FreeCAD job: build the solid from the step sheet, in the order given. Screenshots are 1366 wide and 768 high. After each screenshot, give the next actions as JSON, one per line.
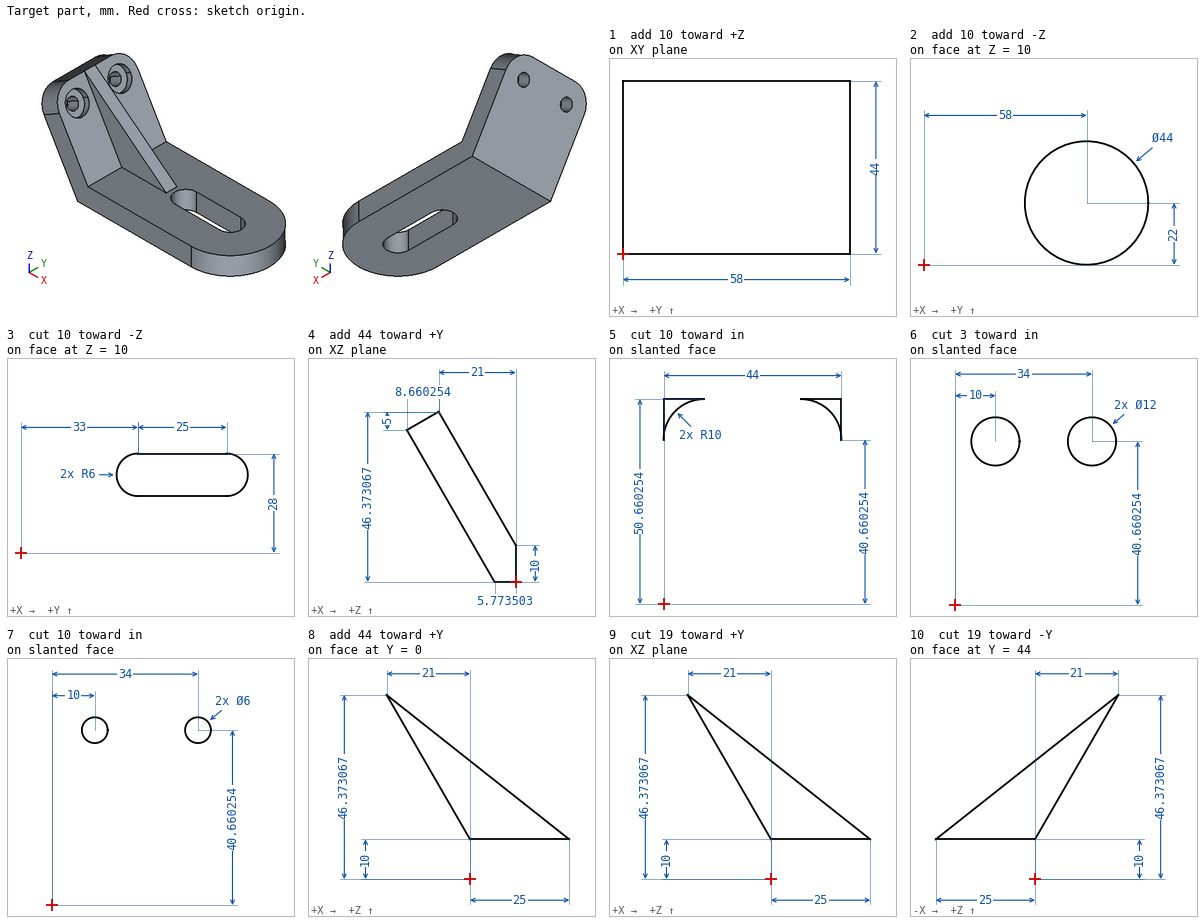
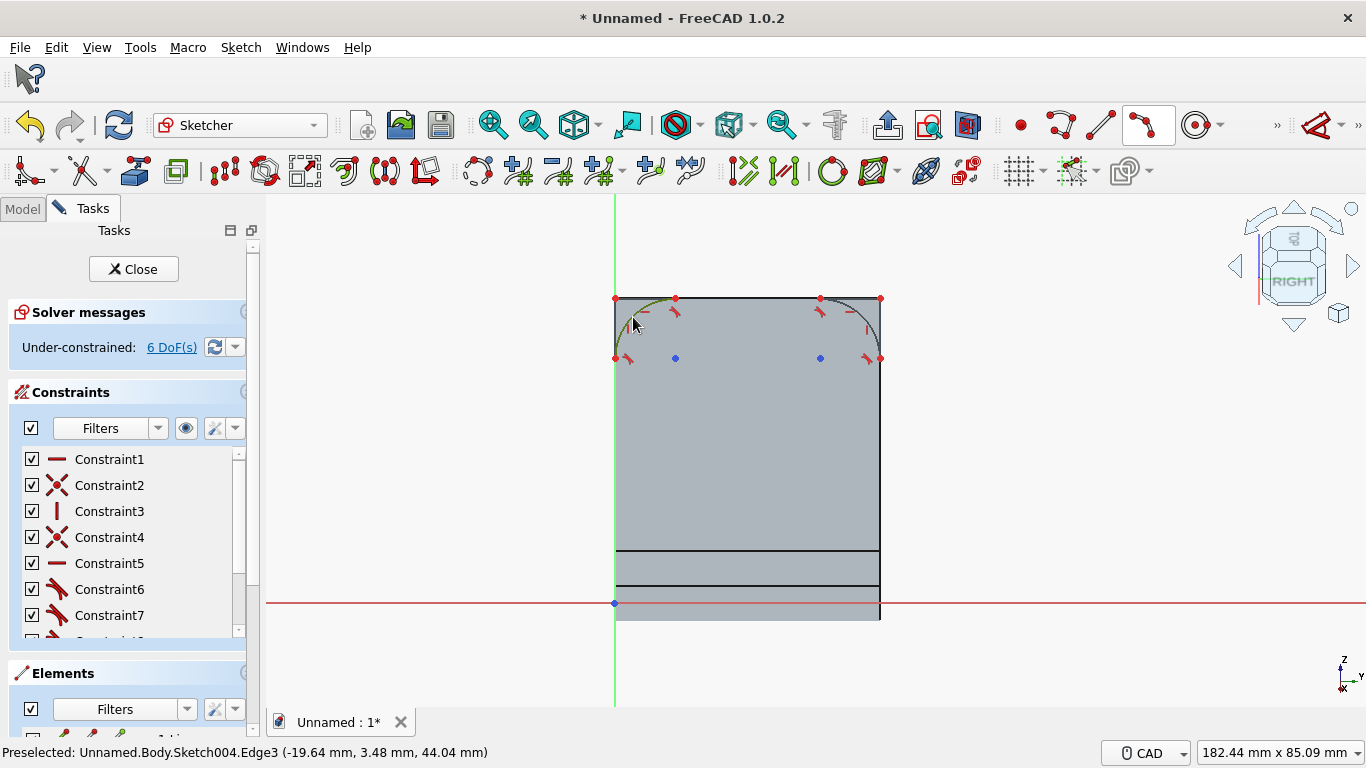
{"action": "left_click", "coordinate": [862, 317]}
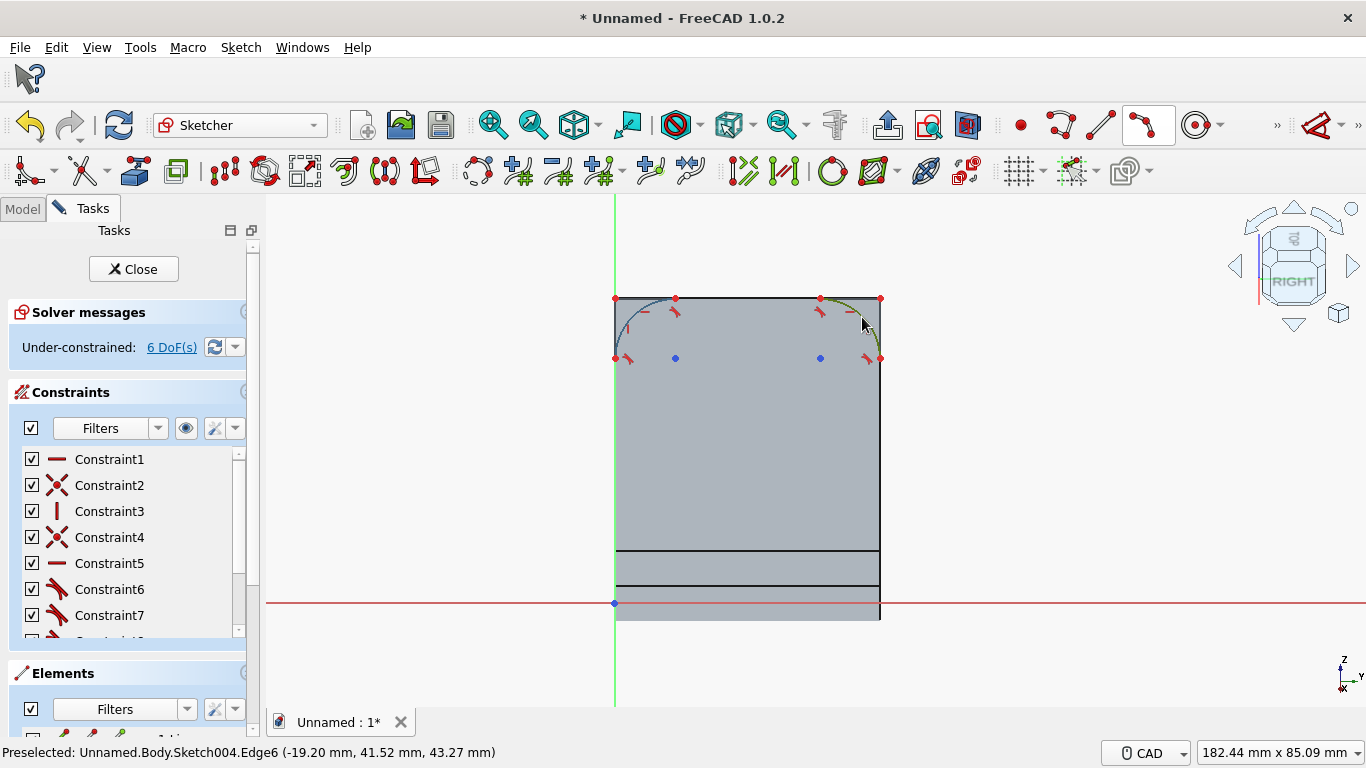
{"action": "key", "text": "e"}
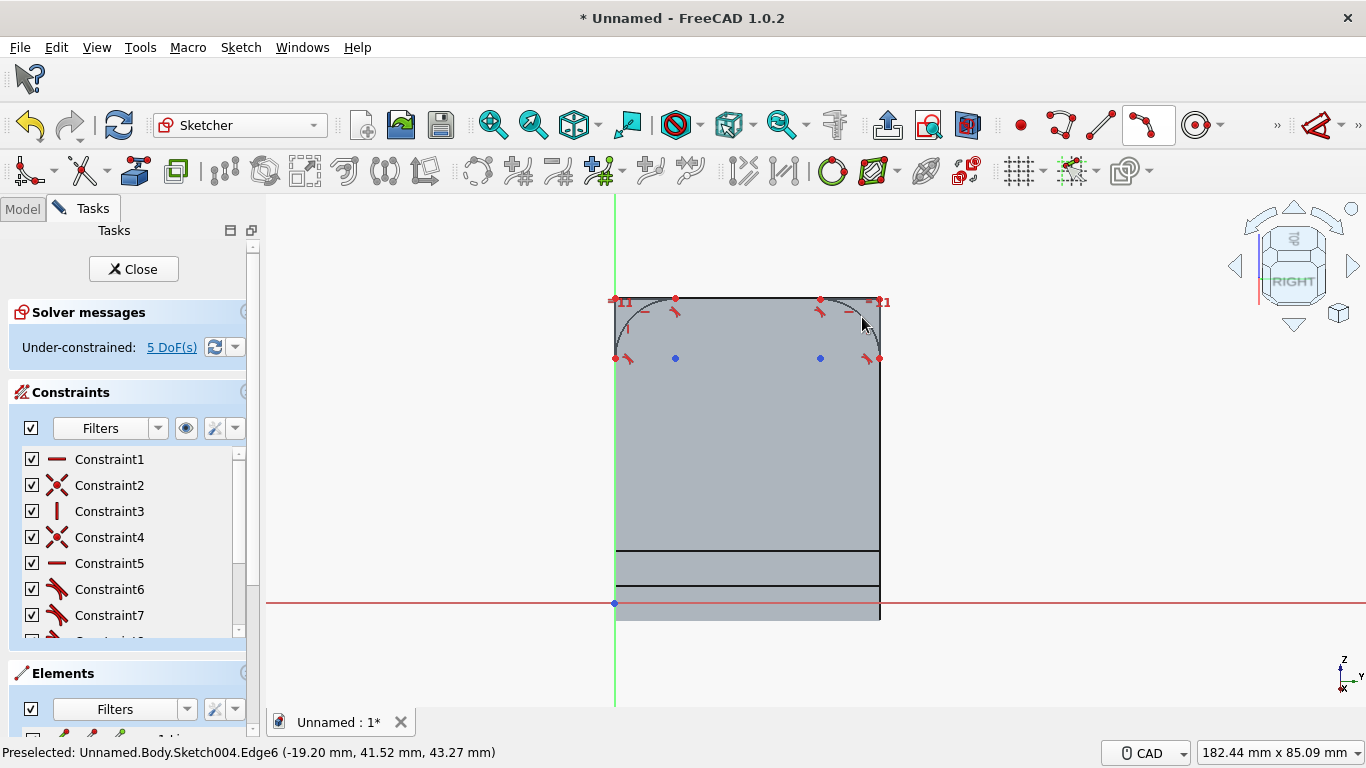
{"action": "left_click", "coordinate": [1316, 126]}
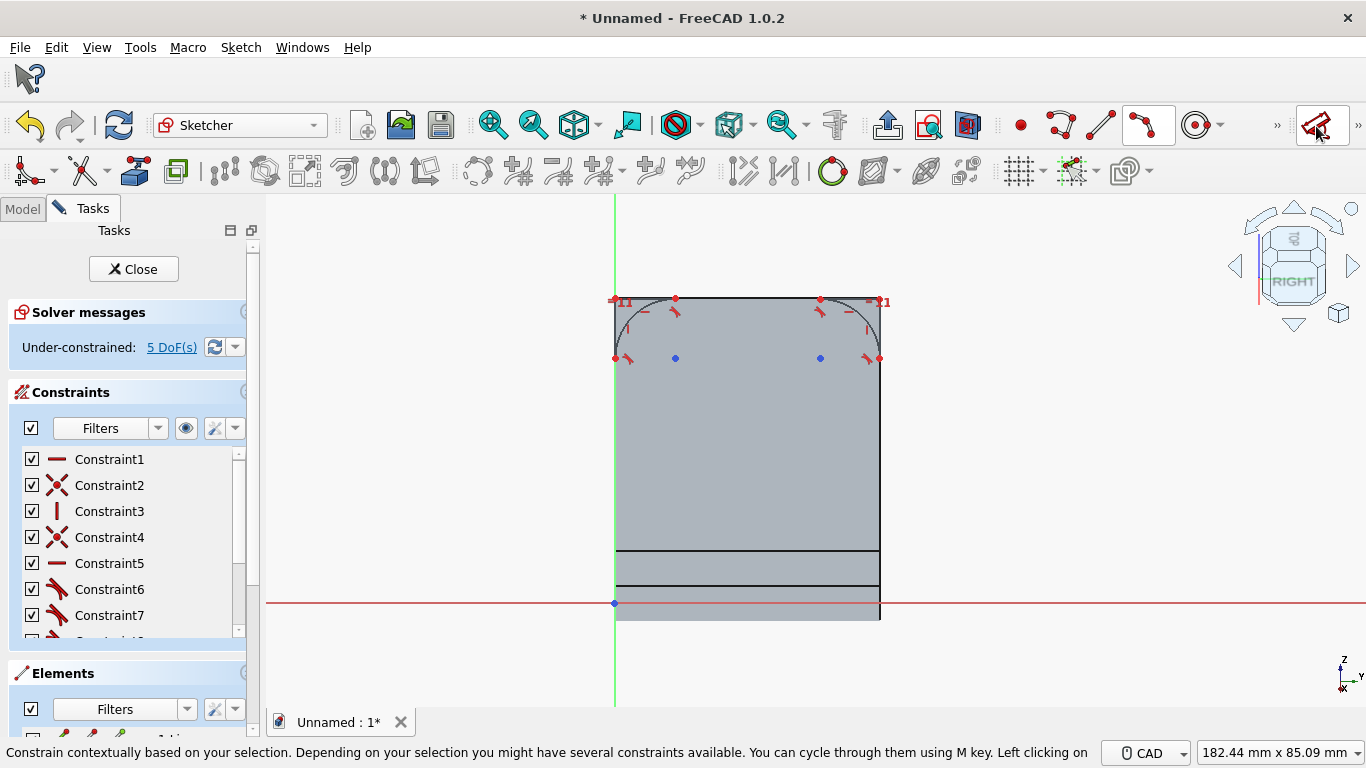
{"action": "left_click", "coordinate": [633, 317]}
{"action": "left_click", "coordinate": [649, 271]}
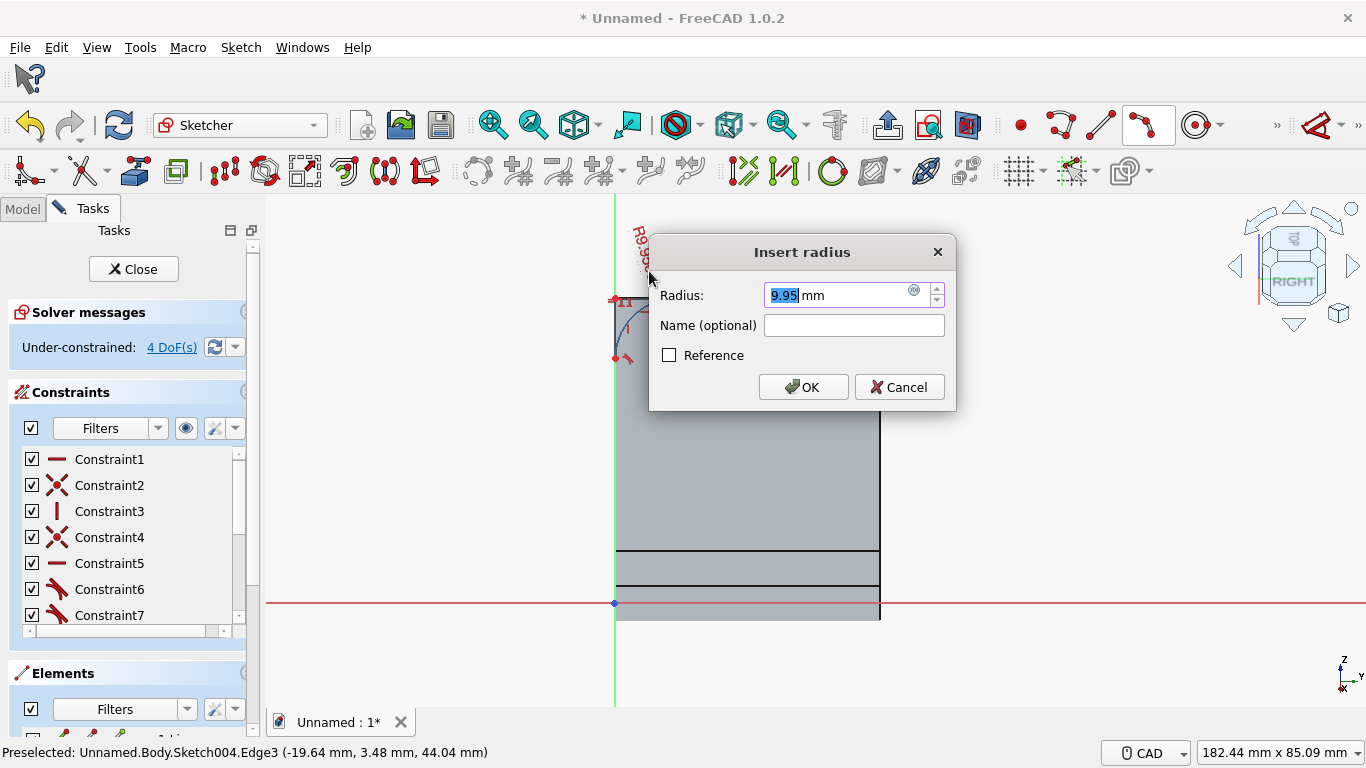
{"action": "type", "text": "10"}
{"action": "key", "text": "Return"}
{"action": "key", "text": "Escape"}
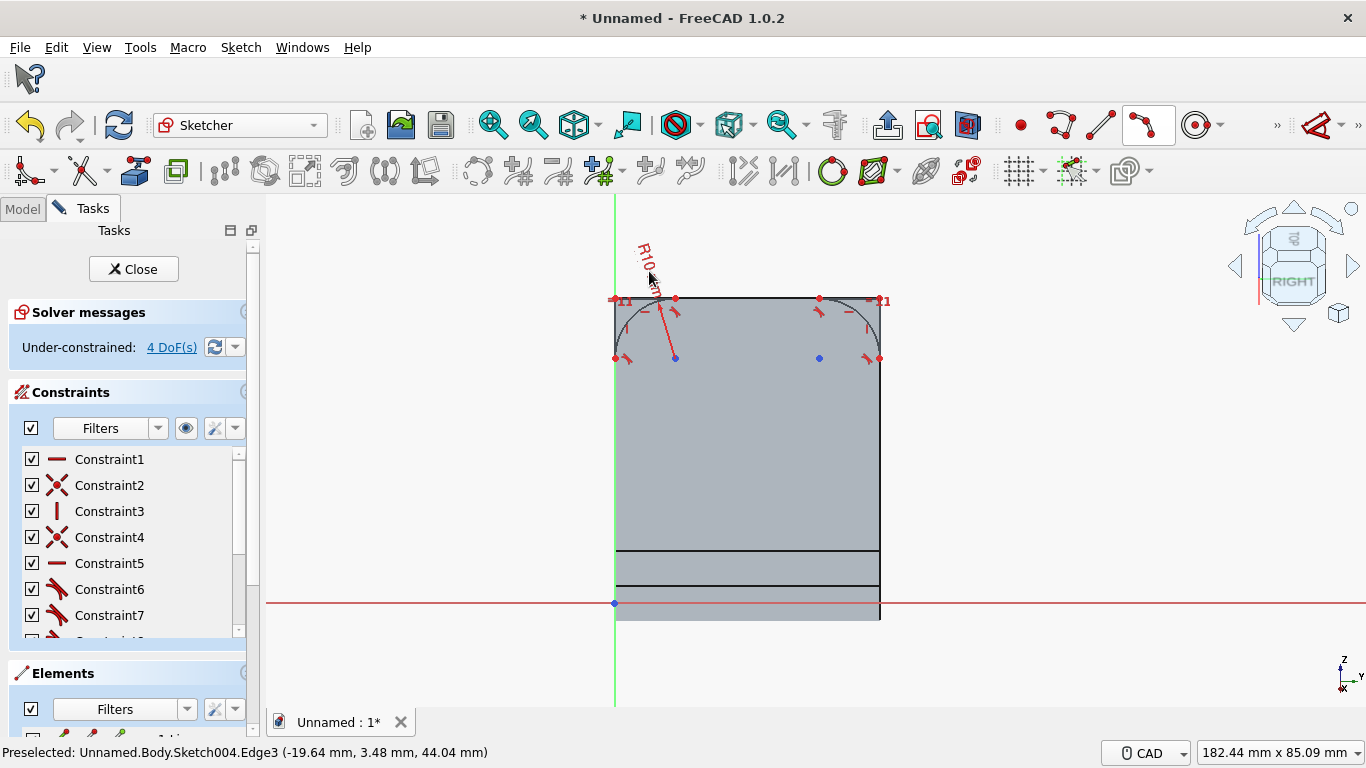
{"action": "left_click", "coordinate": [615, 299]}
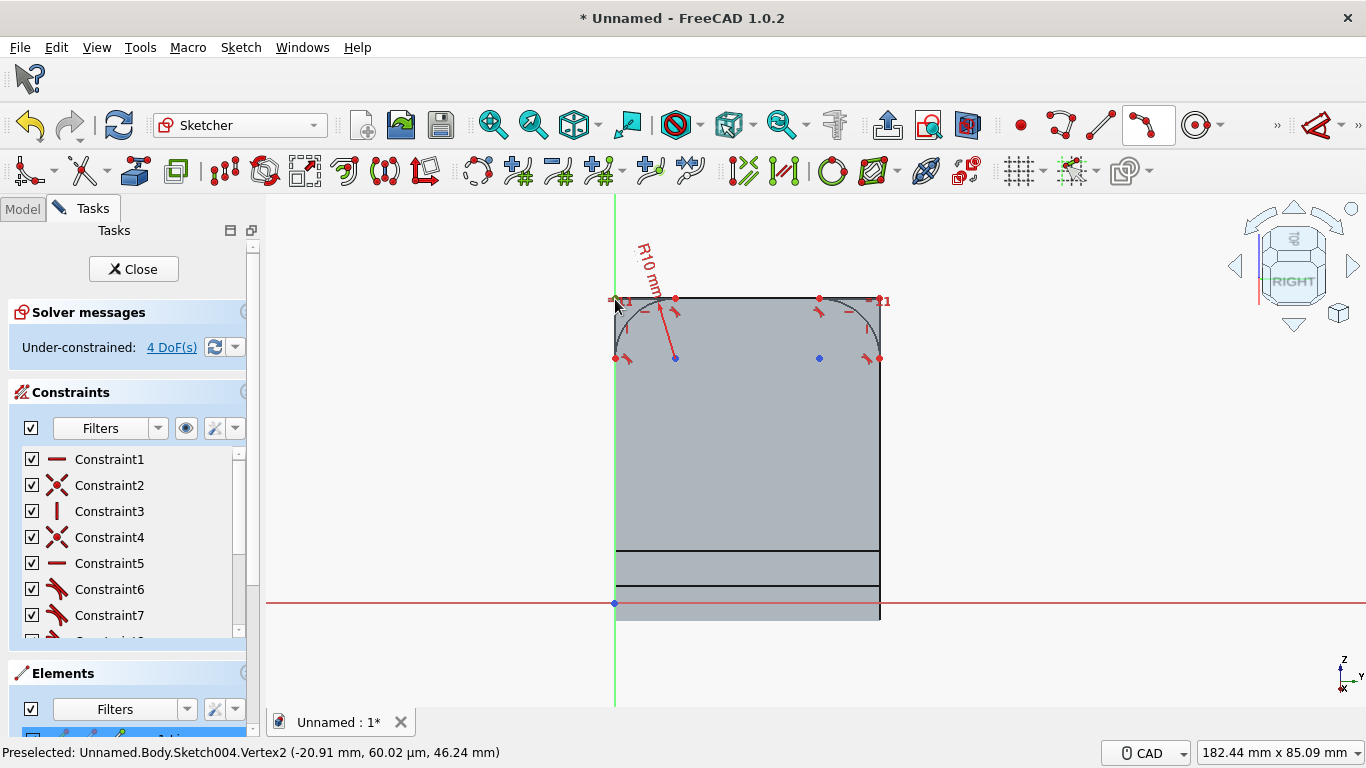
{"action": "left_click", "coordinate": [615, 646]}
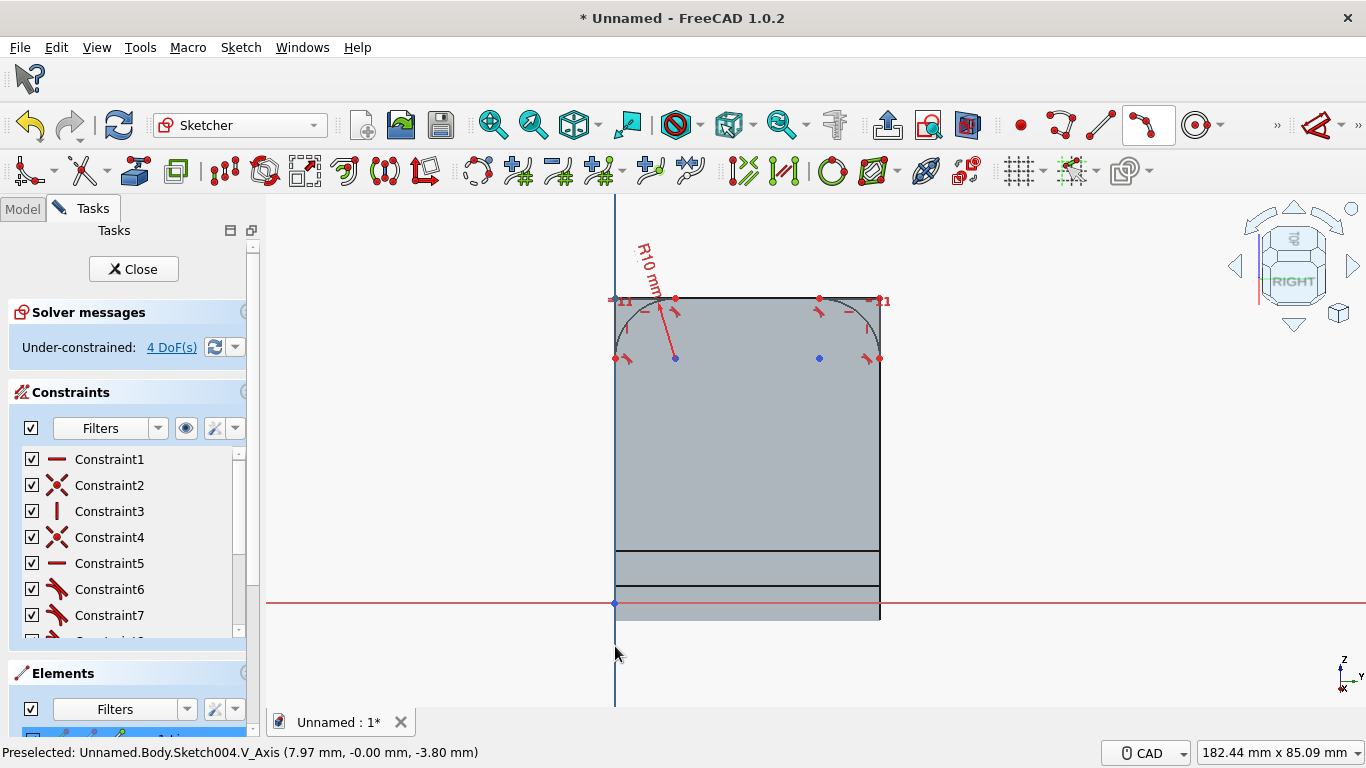
{"action": "key", "text": "c"}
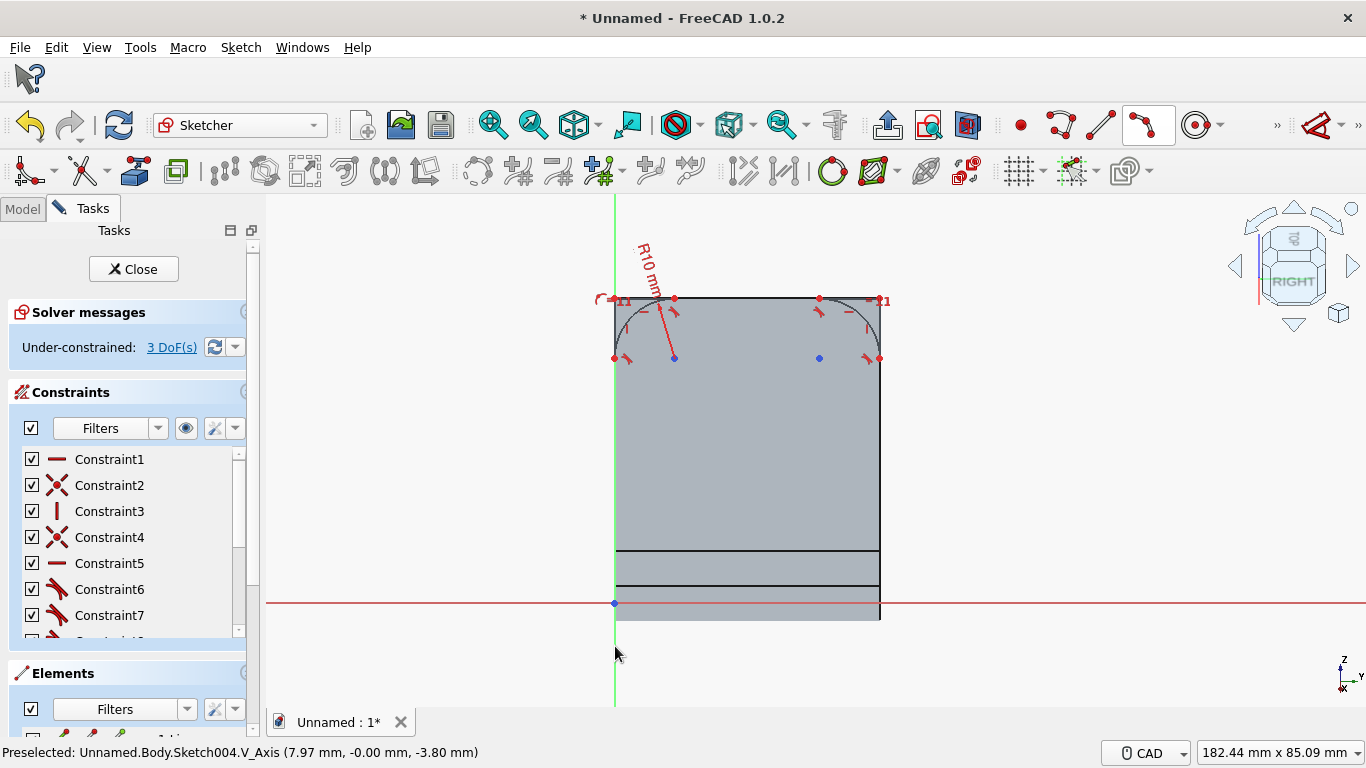
{"action": "left_click", "coordinate": [1316, 126]}